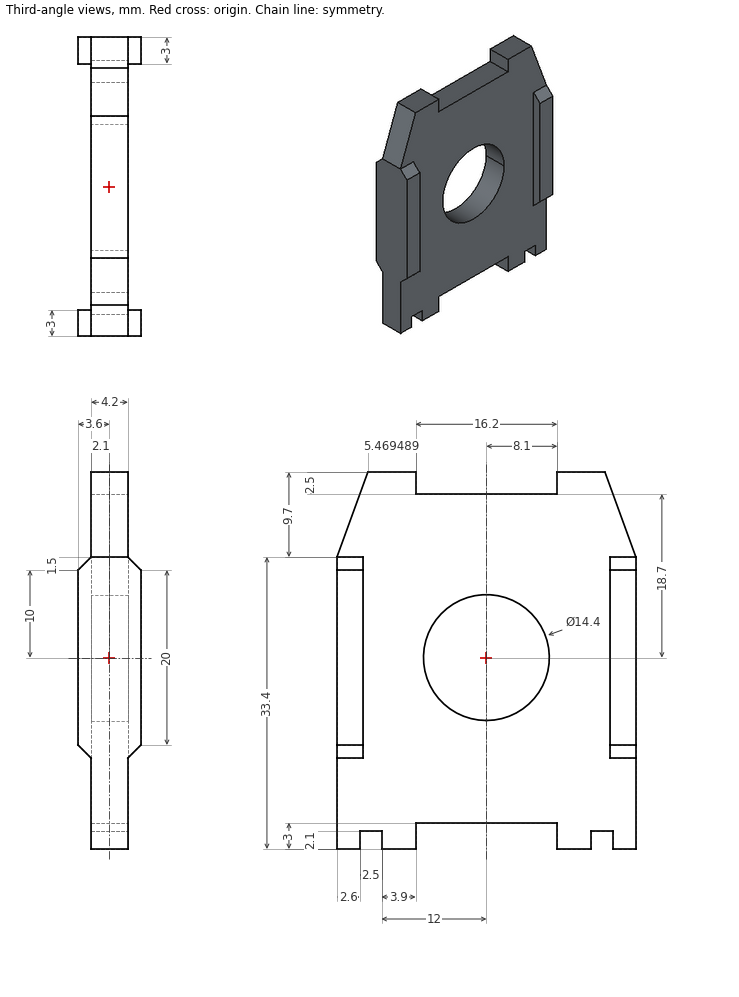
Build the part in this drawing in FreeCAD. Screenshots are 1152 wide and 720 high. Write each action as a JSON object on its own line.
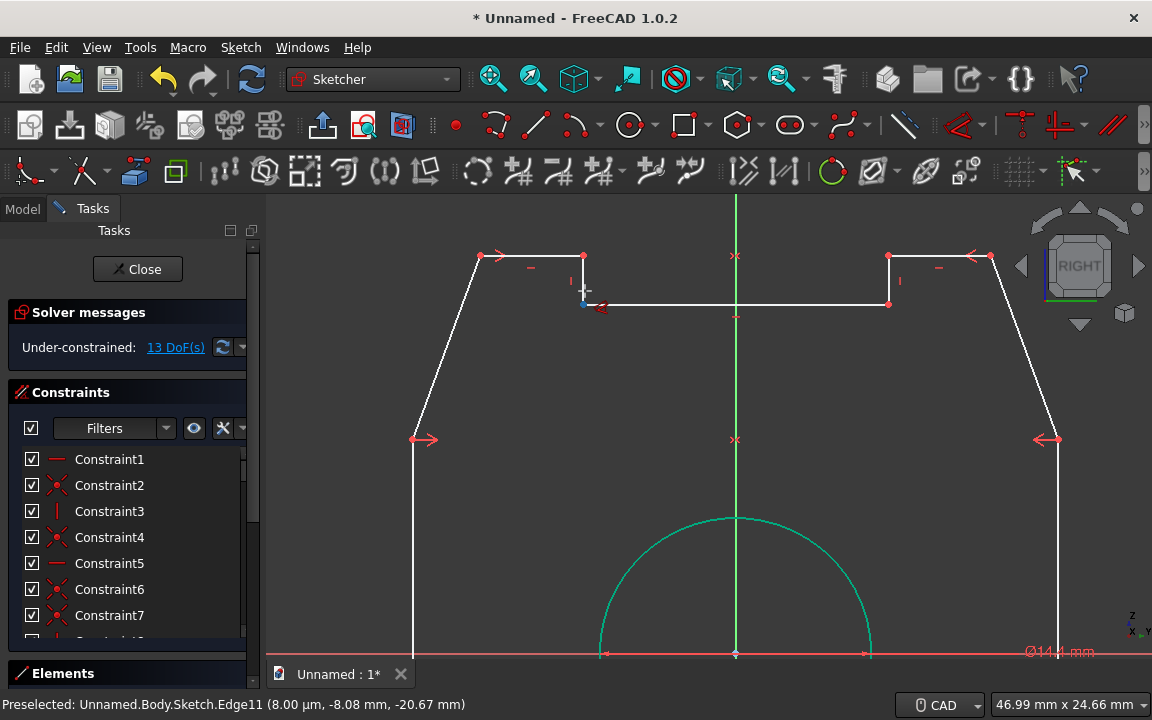
{"action": "left_click", "coordinate": [583, 290]}
{"action": "left_click", "coordinate": [549, 280]}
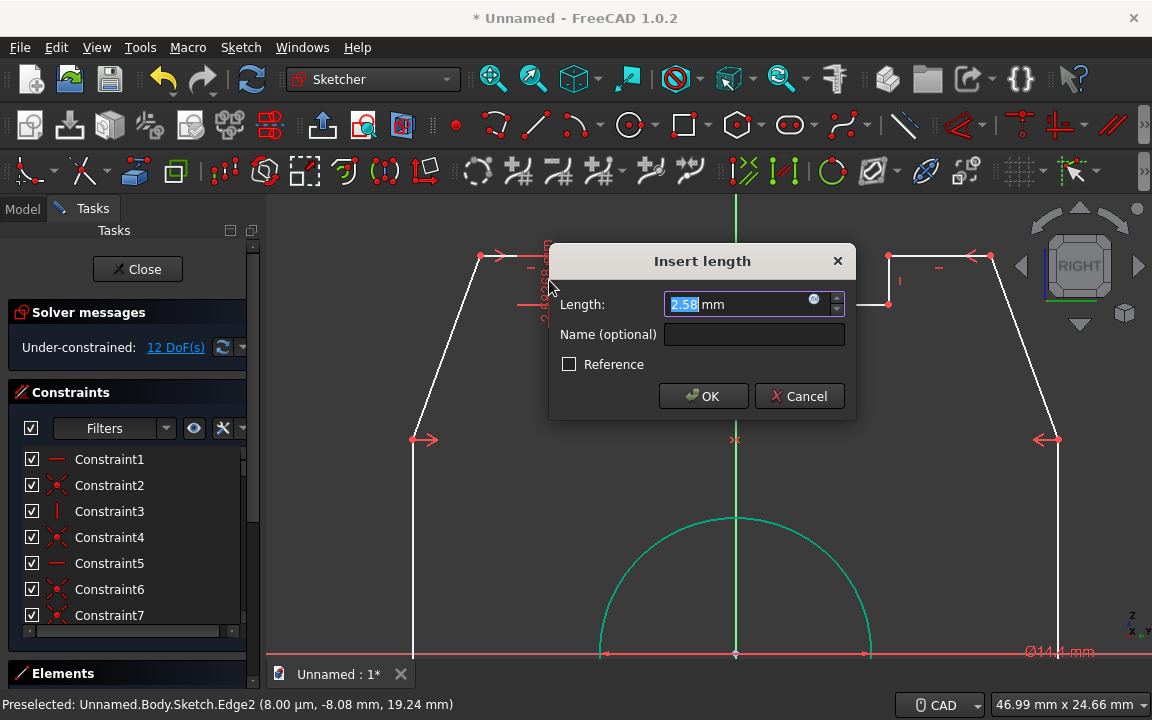
{"action": "type", "text": "2.5"}
{"action": "key", "text": "Return"}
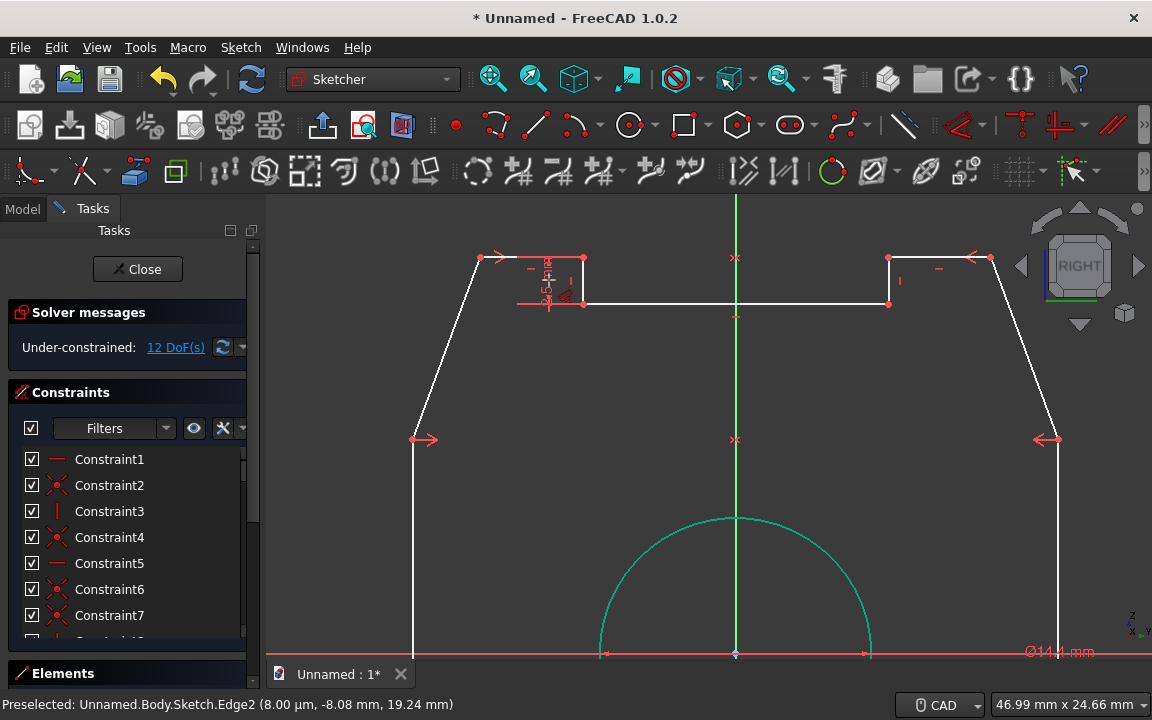
{"action": "scroll", "coordinate": [585, 290], "scroll_direction": "down", "scroll_amount": 5}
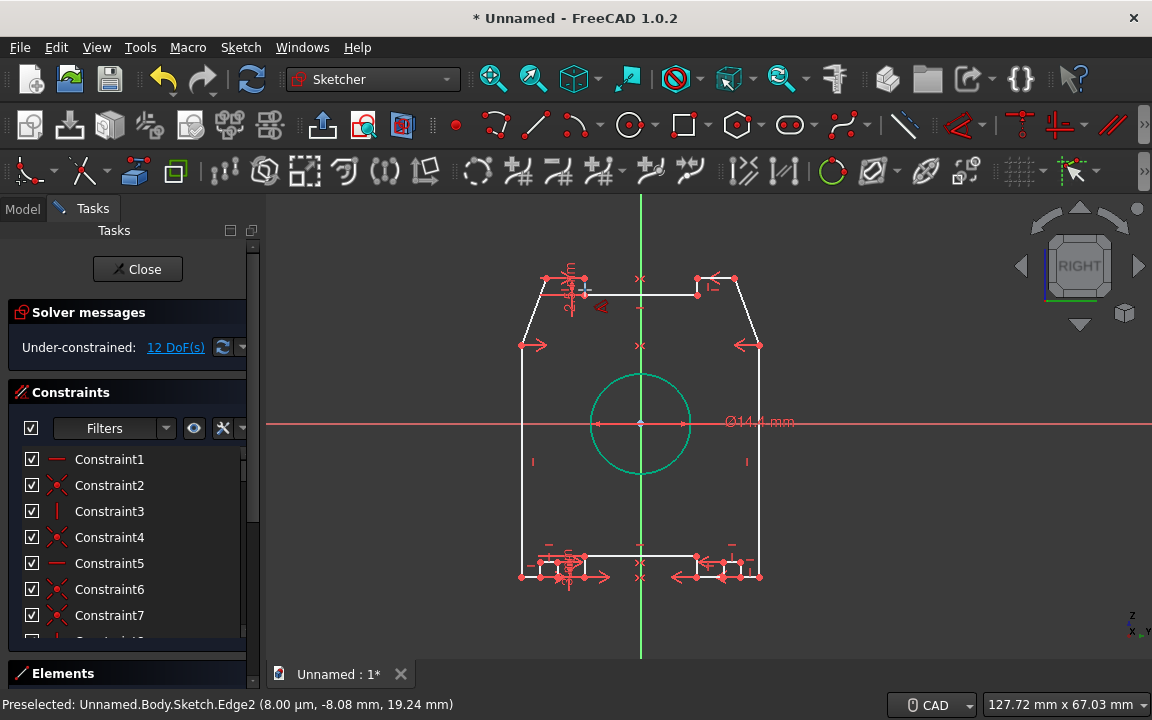
{"action": "scroll", "coordinate": [527, 577], "scroll_direction": "up", "scroll_amount": 5}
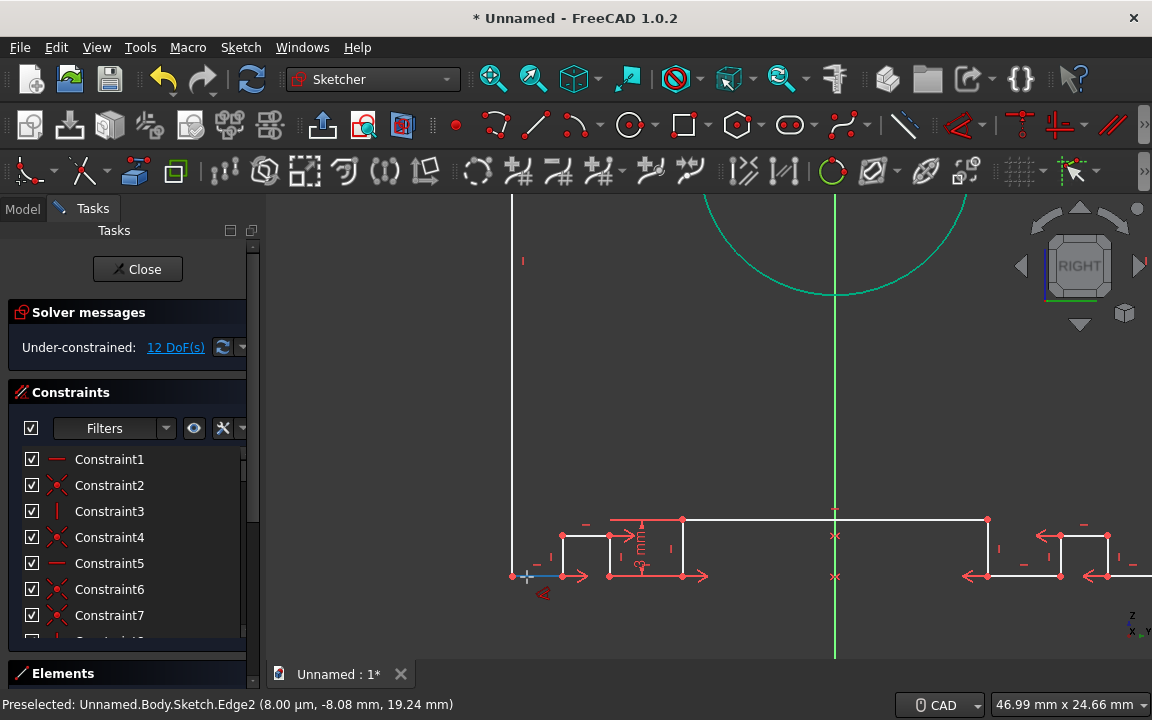
{"action": "left_click", "coordinate": [527, 576]}
{"action": "left_click", "coordinate": [538, 610]}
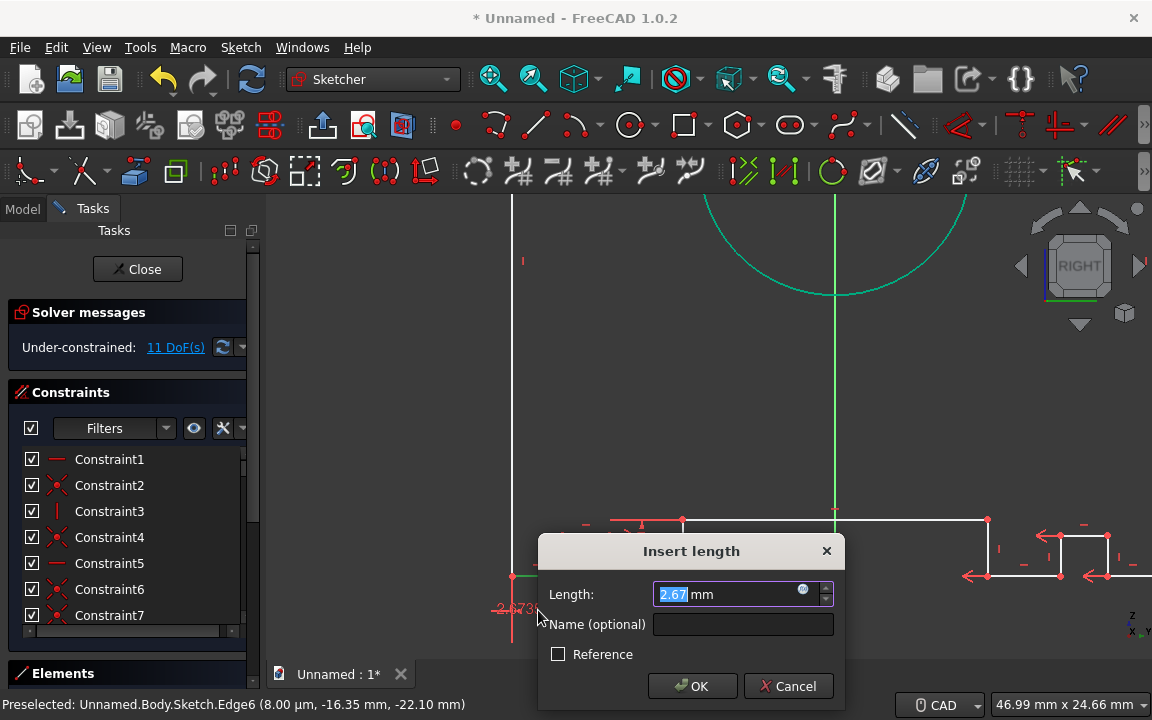
{"action": "type", "text": "2.6"}
{"action": "key", "text": "Return"}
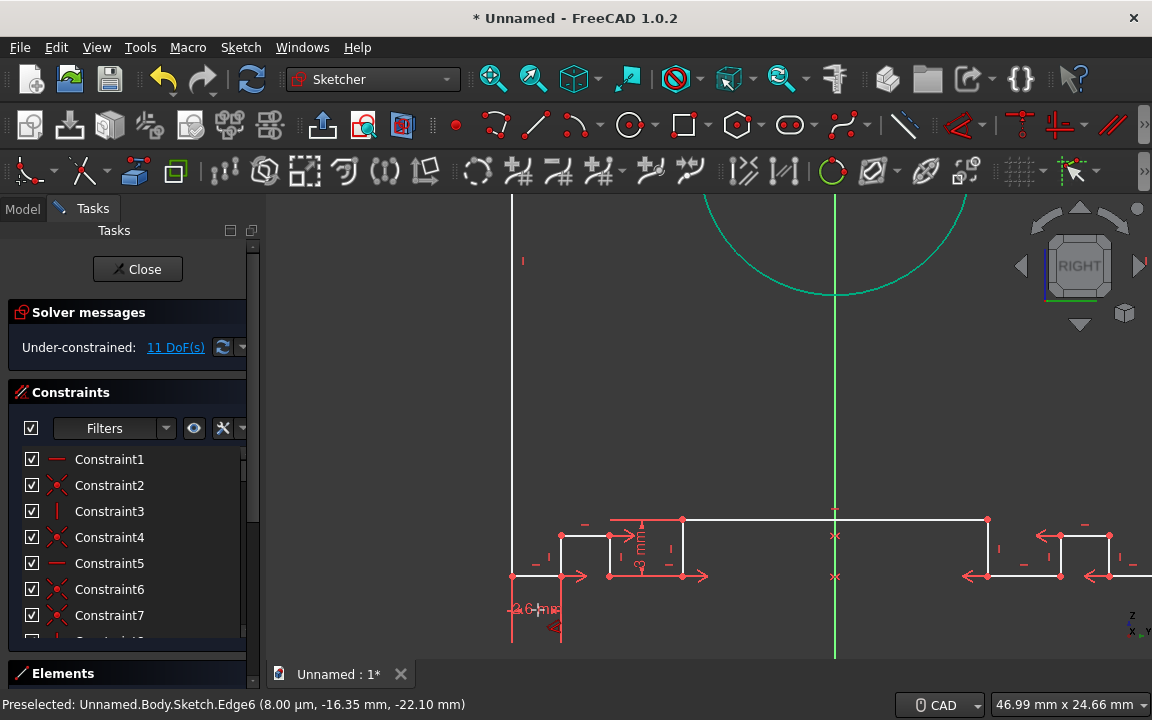
{"action": "left_click", "coordinate": [561, 564]}
{"action": "left_click", "coordinate": [527, 556]}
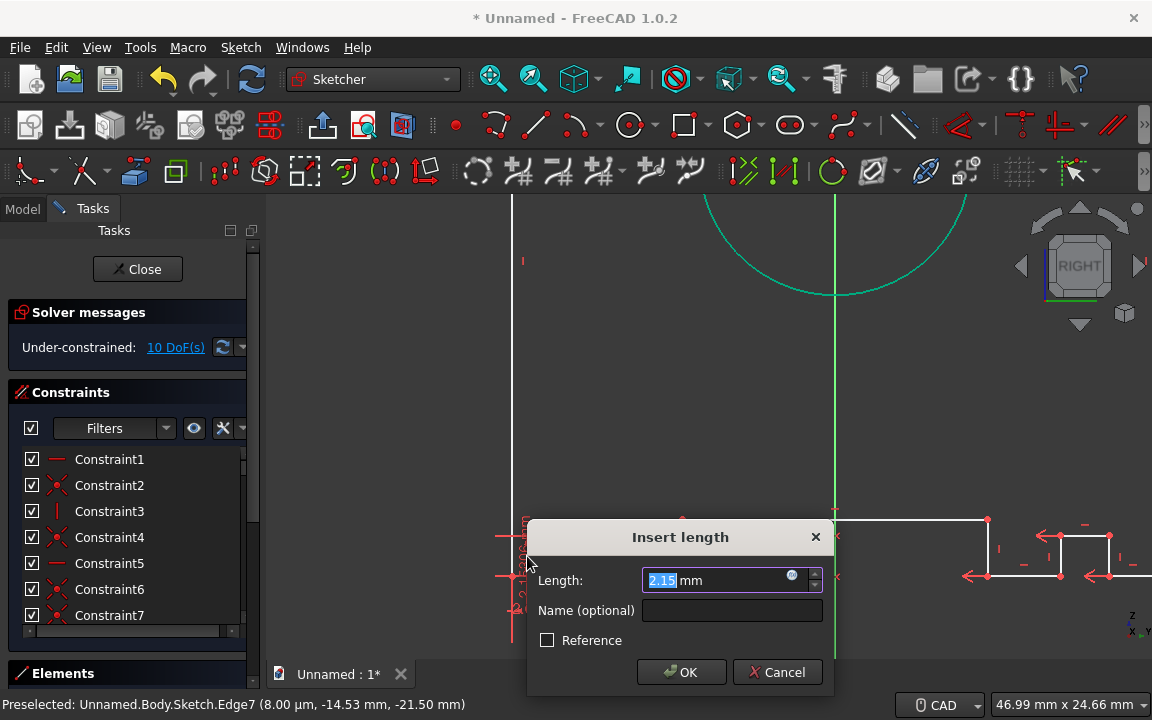
{"action": "type", "text": "2.1"}
{"action": "key", "text": "Return"}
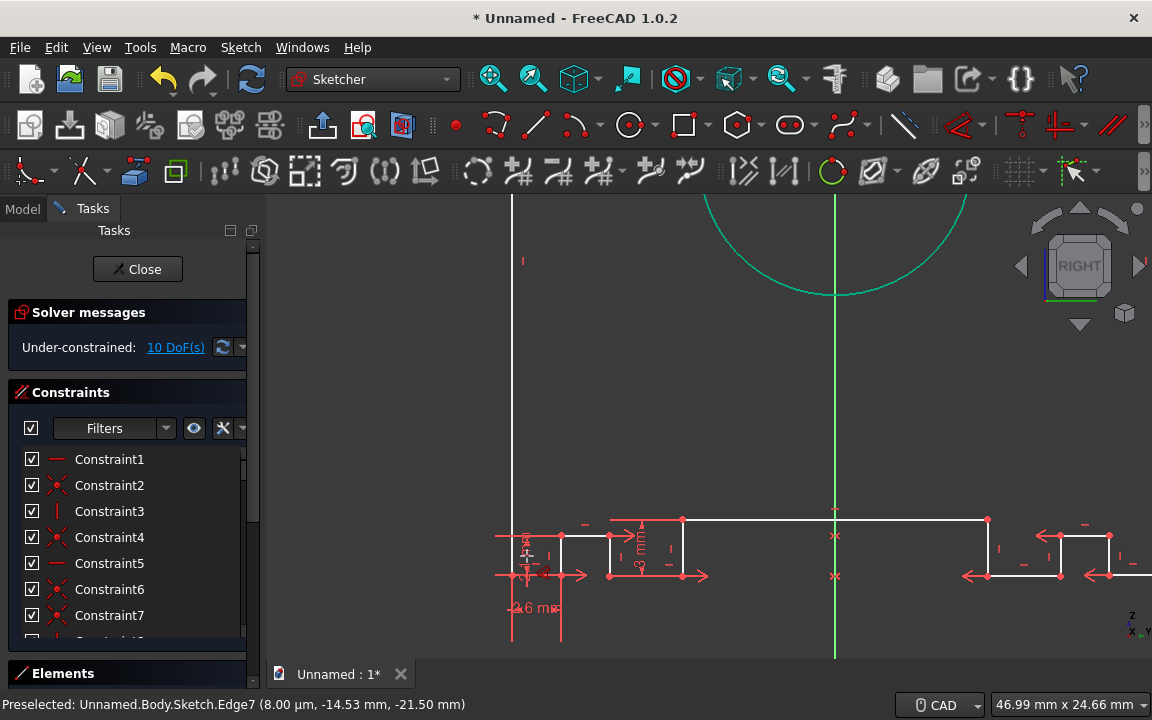
{"action": "left_click", "coordinate": [576, 536]}
{"action": "left_click", "coordinate": [586, 502]}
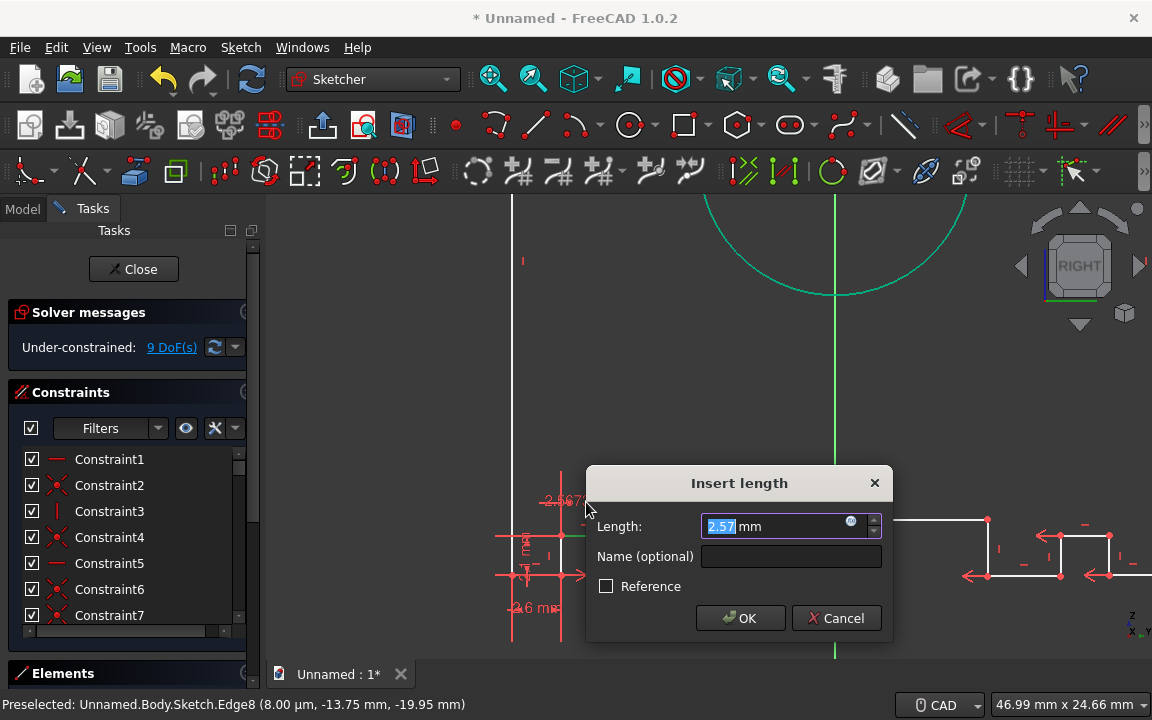
{"action": "type", "text": "2.5"}
{"action": "key", "text": "Return"}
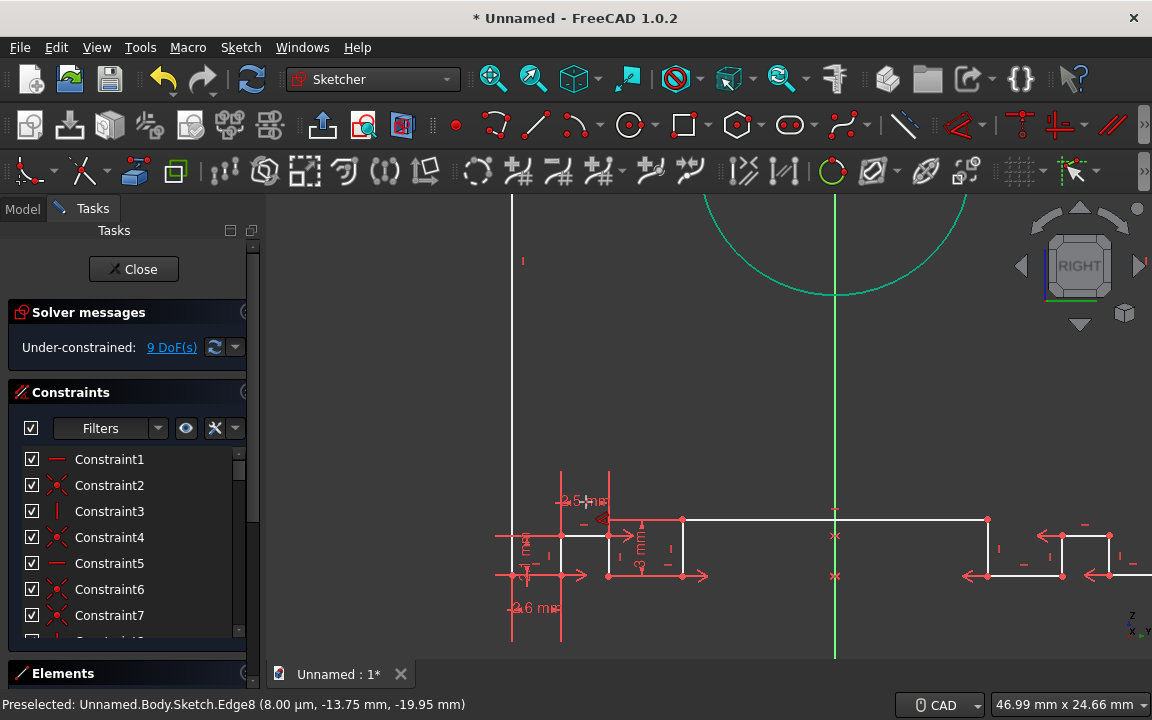
{"action": "left_click", "coordinate": [609, 548]}
{"action": "left_click", "coordinate": [715, 556]}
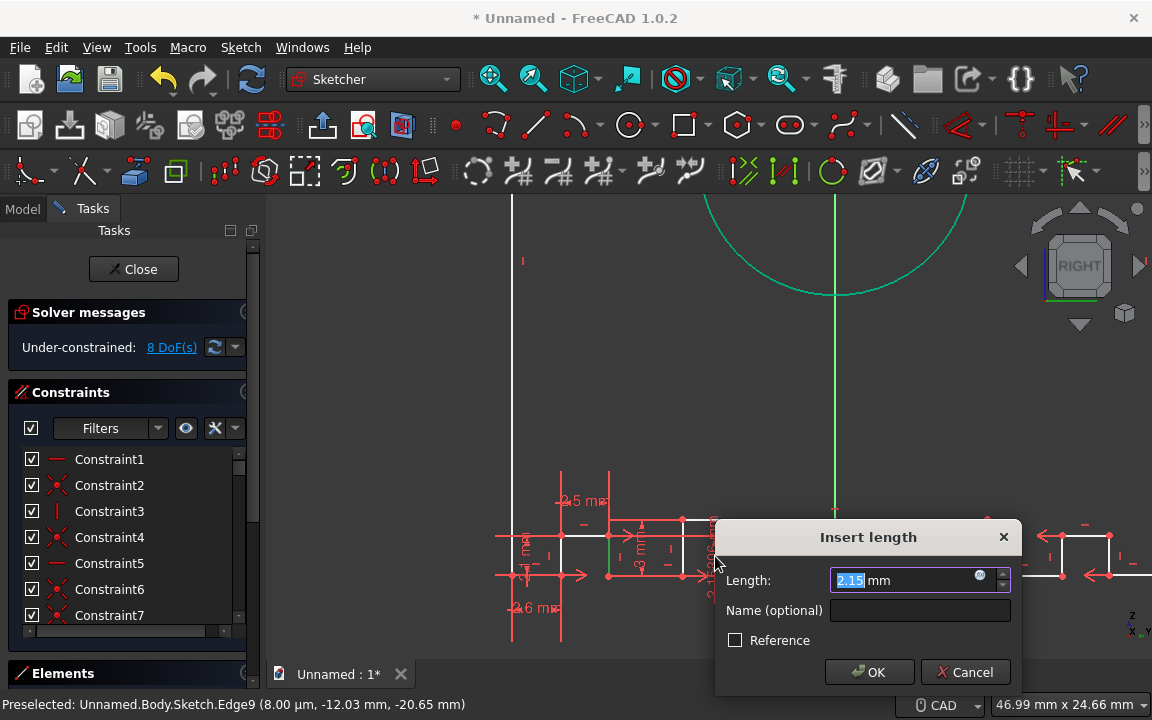
{"action": "type", "text": "2.1"}
{"action": "key", "text": "Return"}